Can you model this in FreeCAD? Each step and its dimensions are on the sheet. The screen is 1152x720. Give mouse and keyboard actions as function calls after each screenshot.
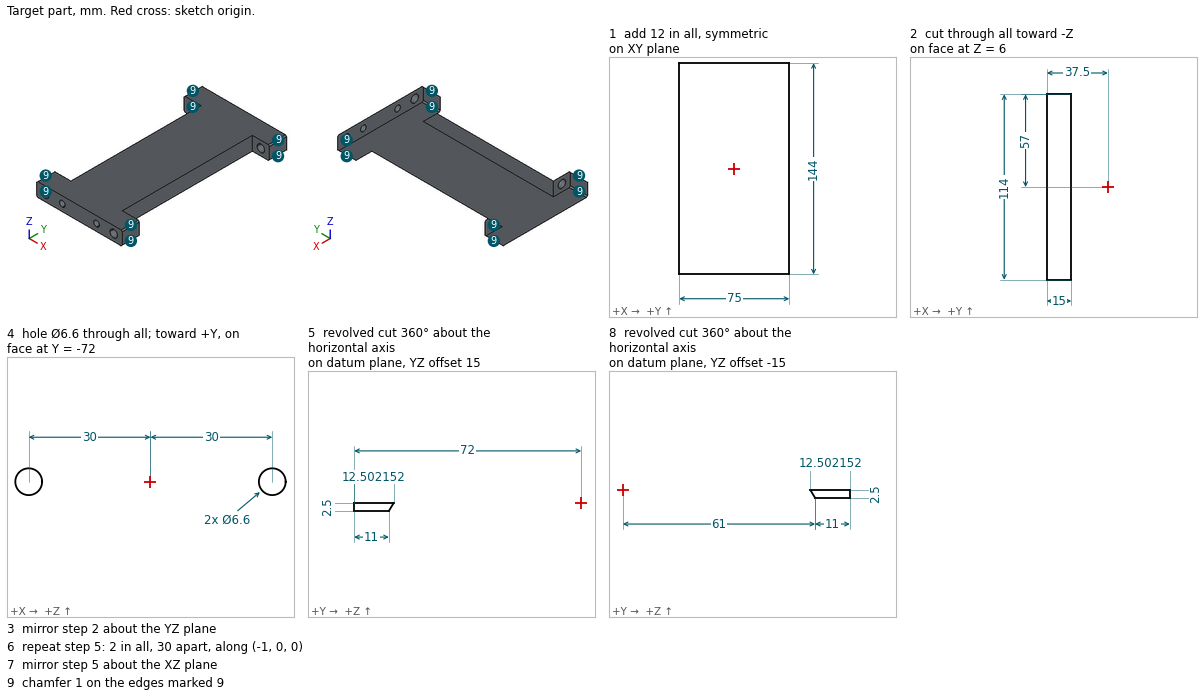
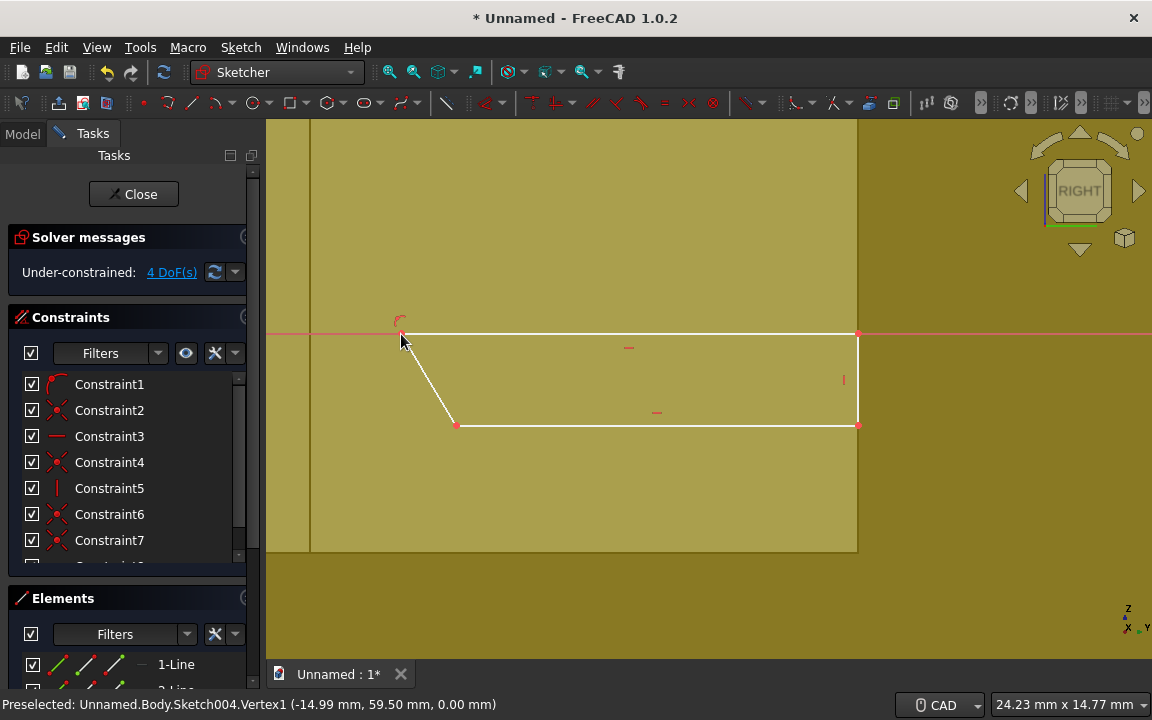
click(486, 104)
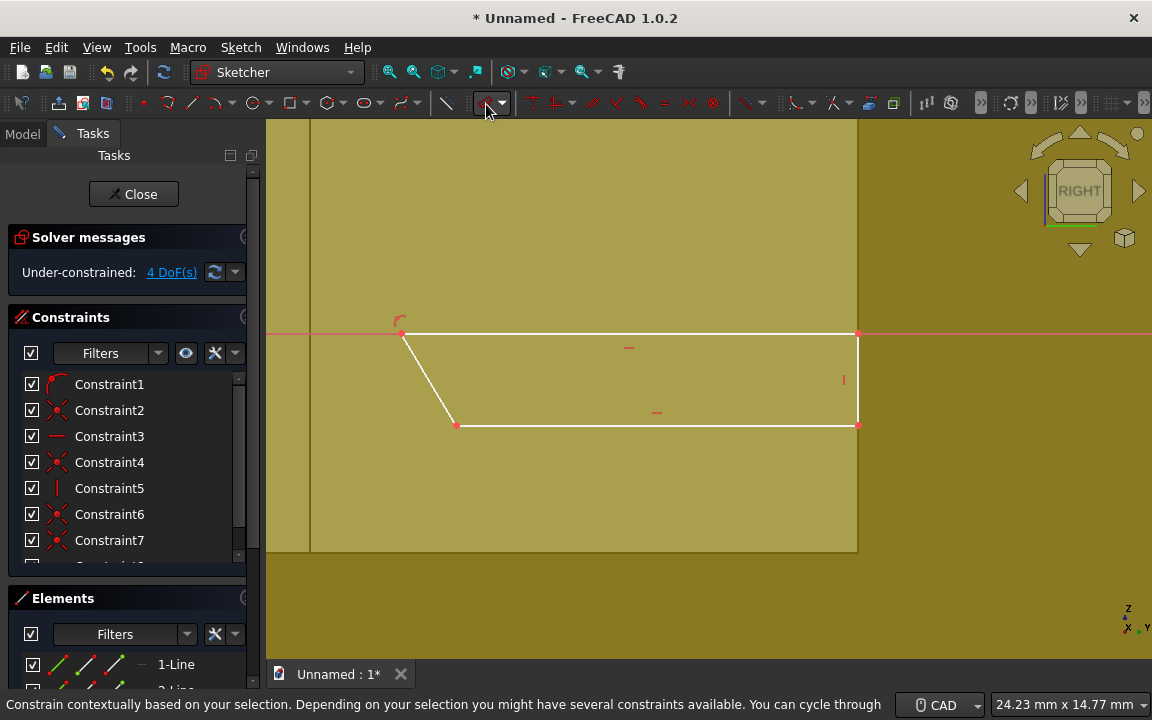
click(577, 426)
click(657, 460)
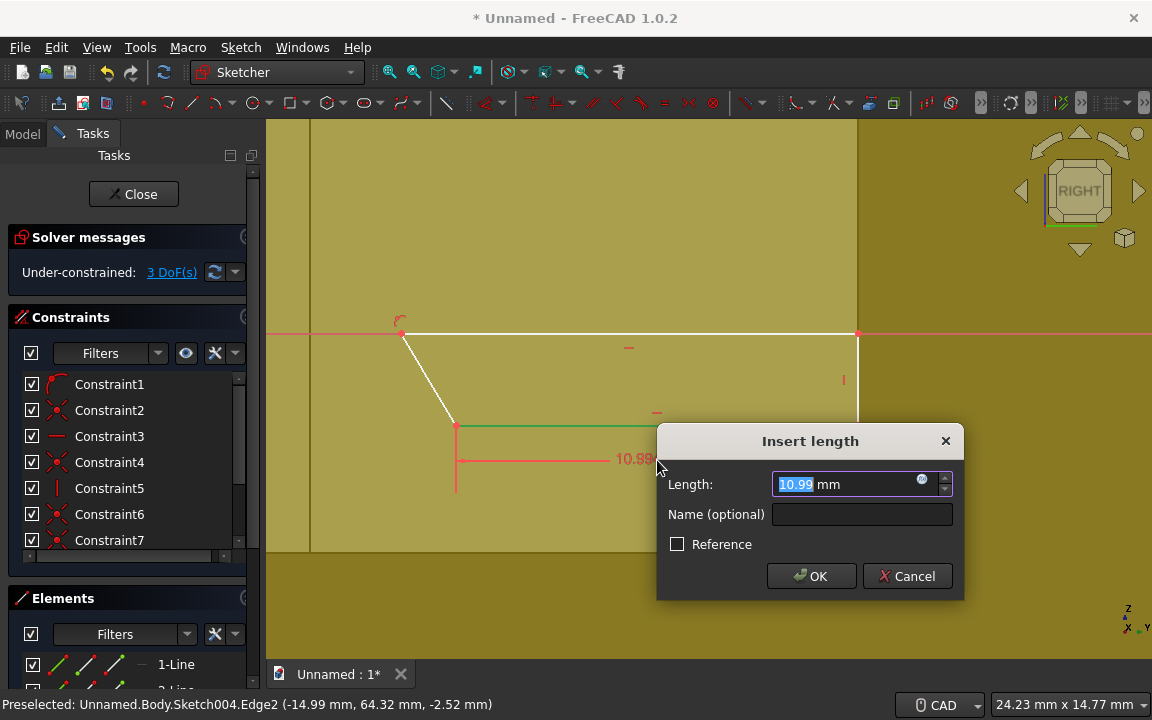
text(11)
key(Return)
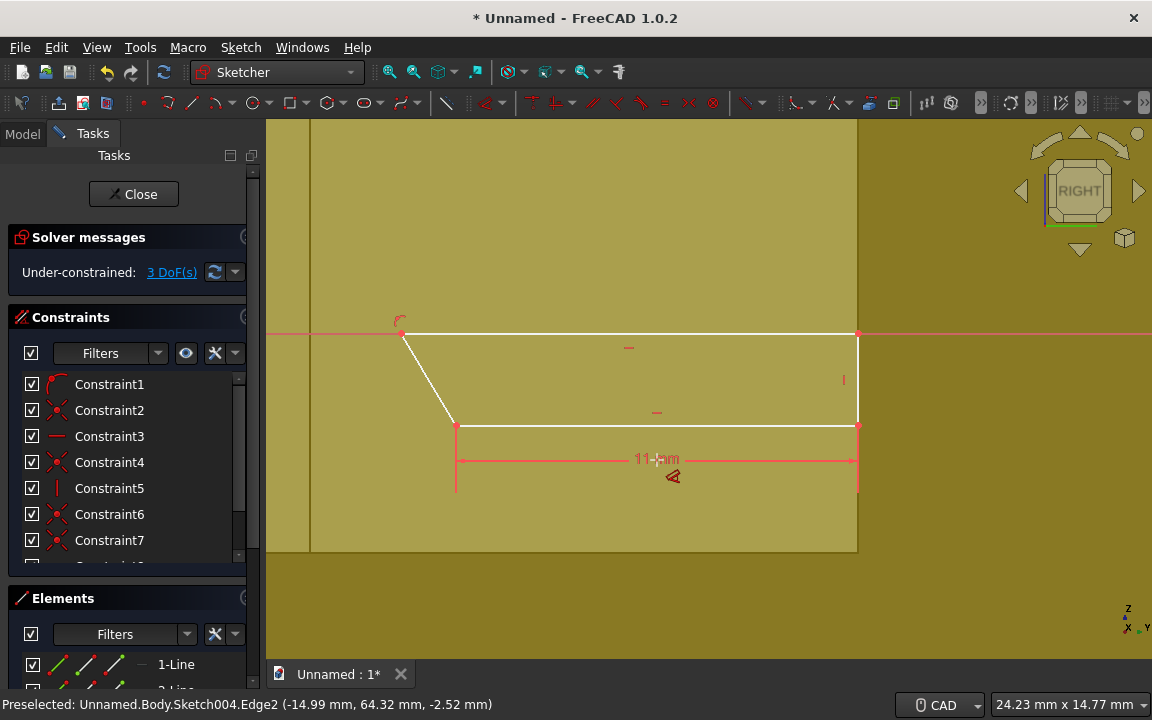
click(858, 398)
click(892, 380)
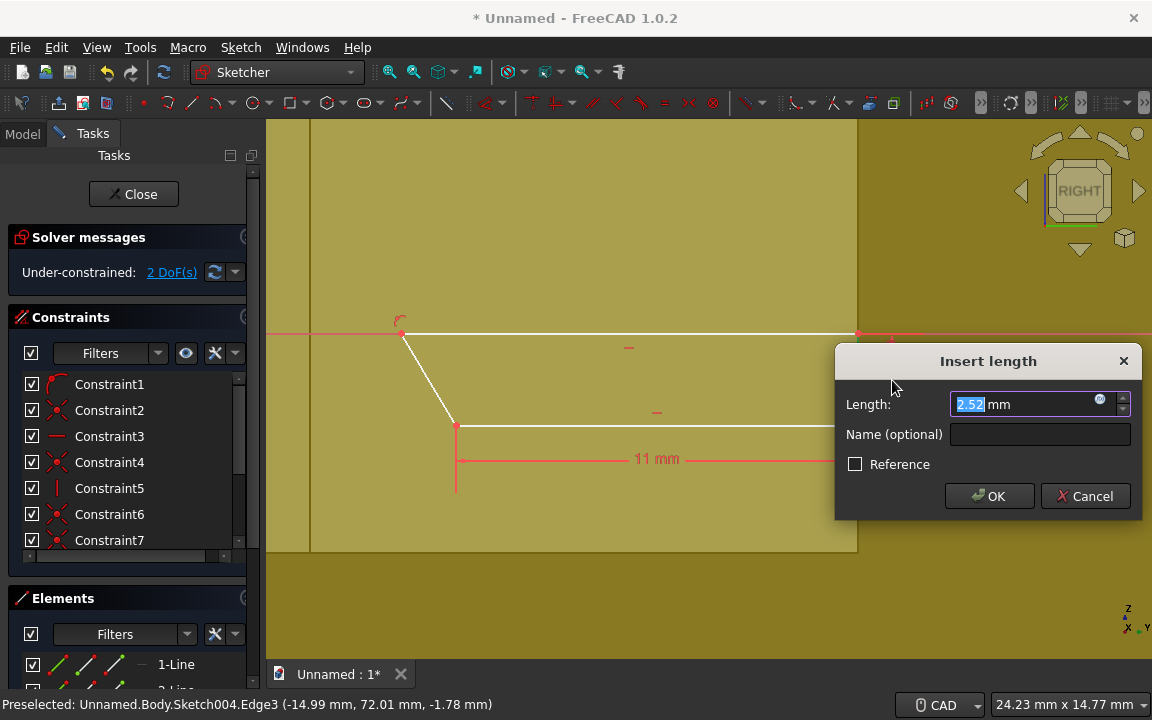
text(2.5)
key(Return)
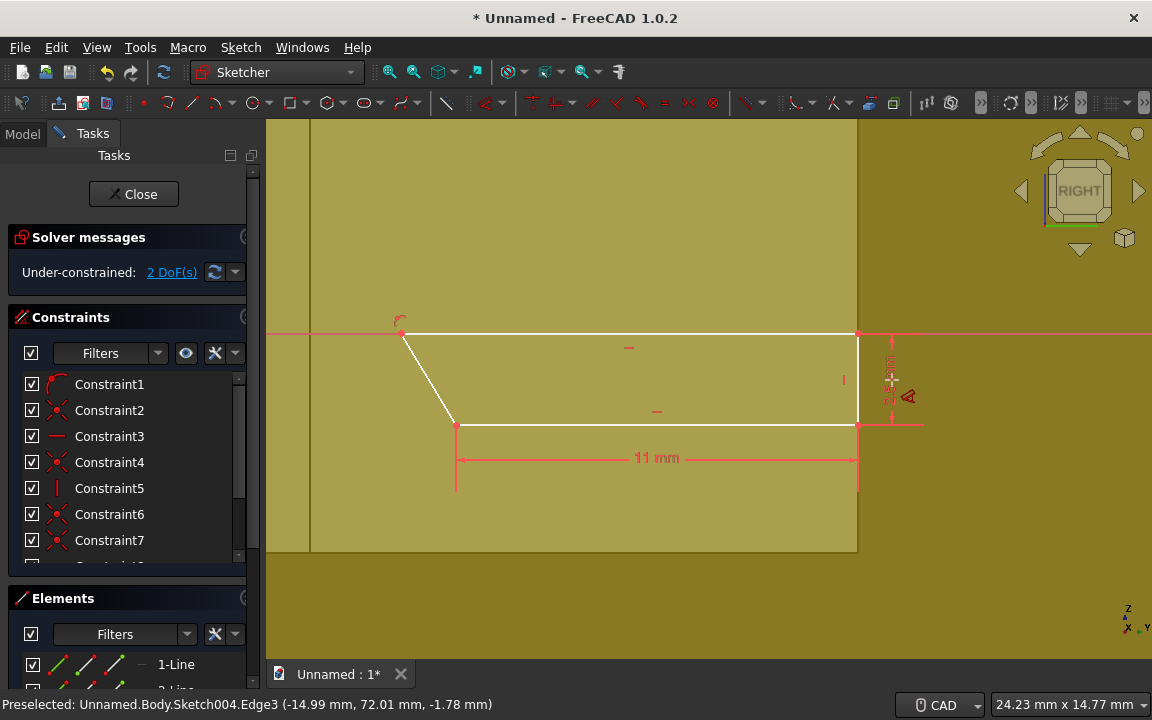
click(456, 425)
click(375, 459)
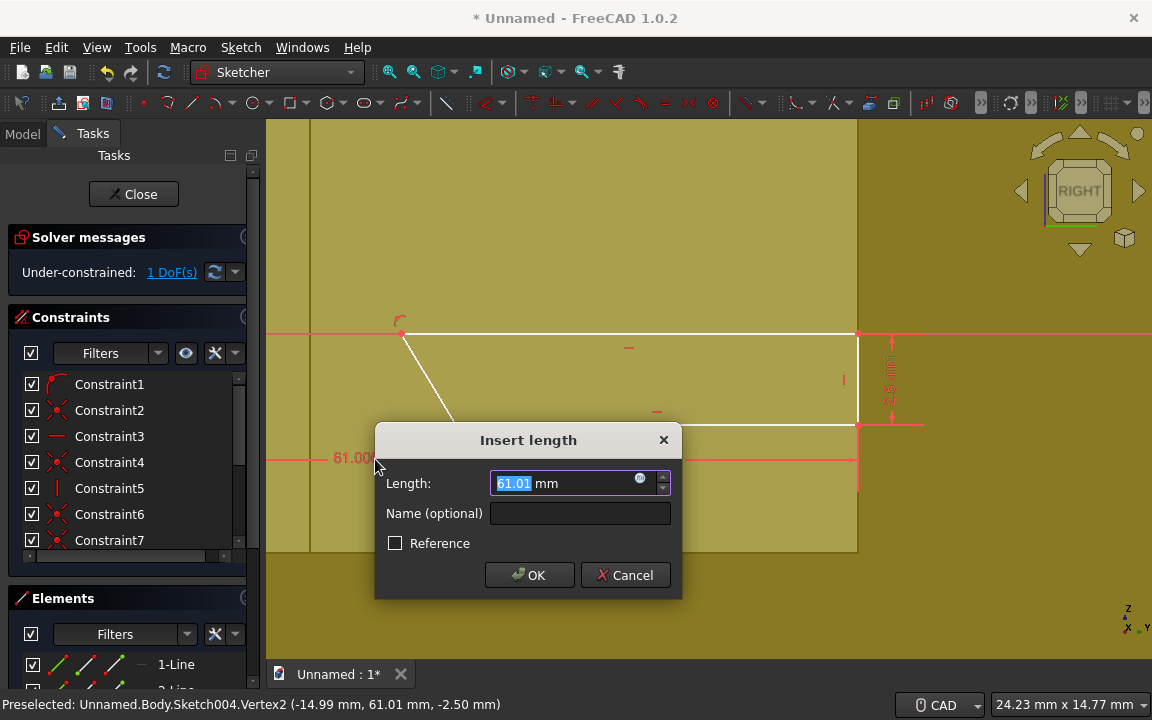
text(61)
key(Return)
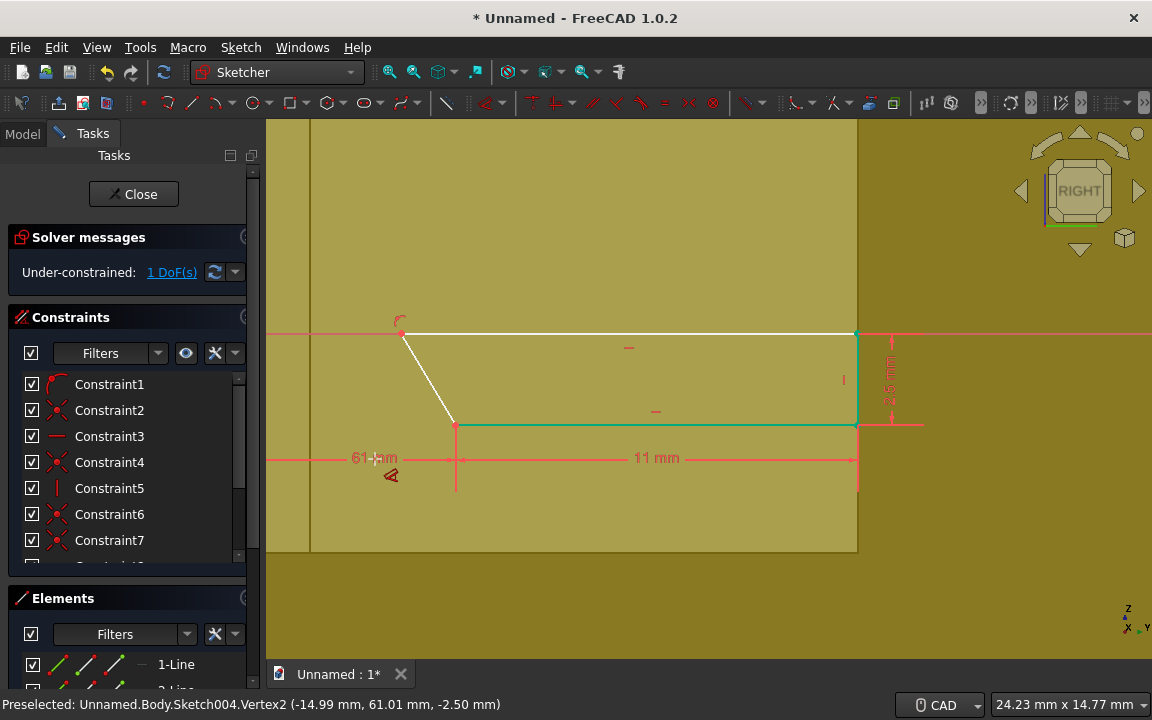
click(721, 334)
click(629, 300)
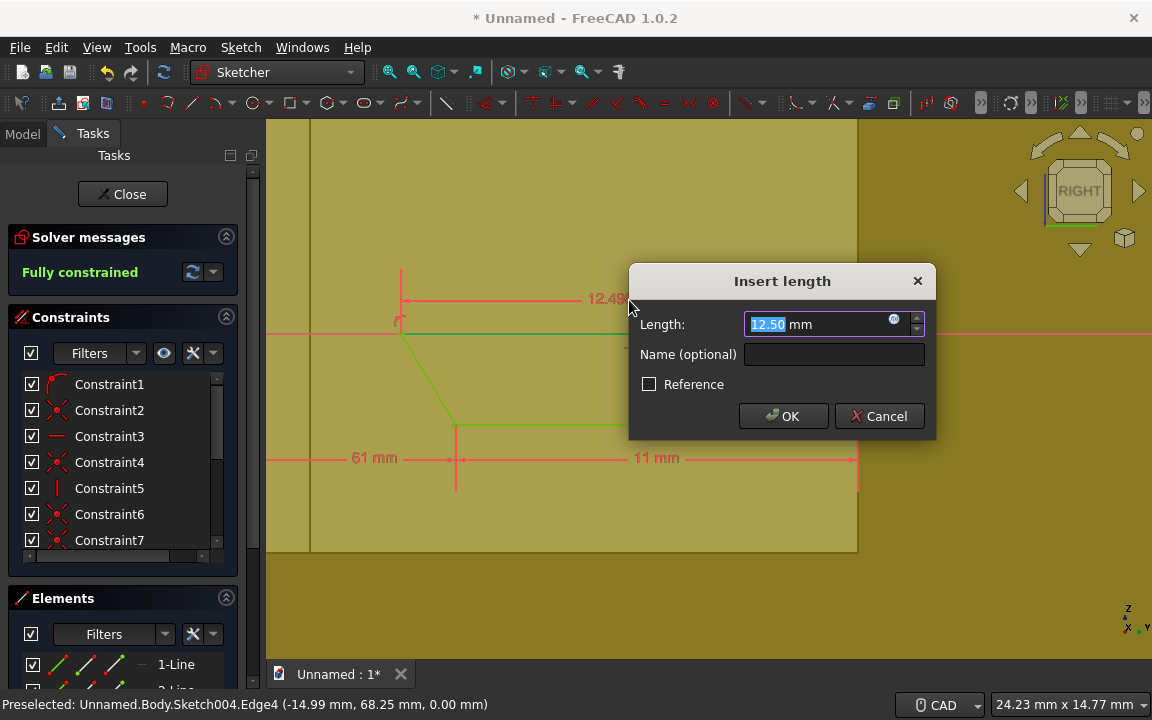
text(12.502152)
key(Return)
key(Escape)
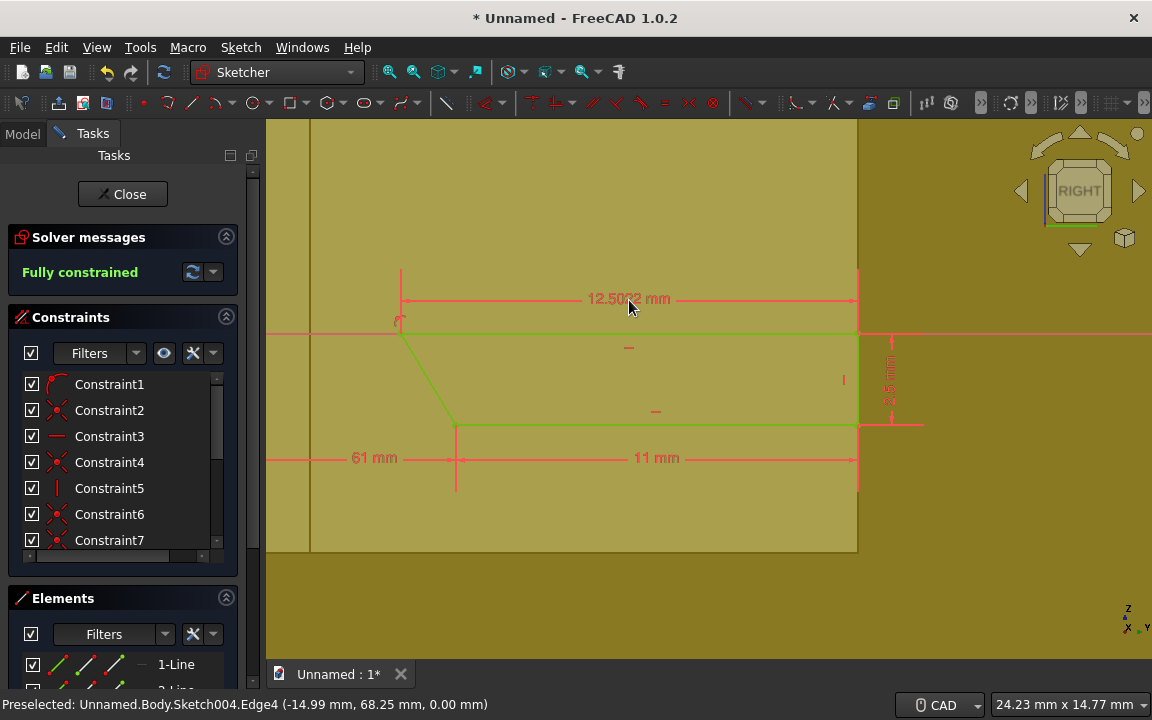
click(123, 194)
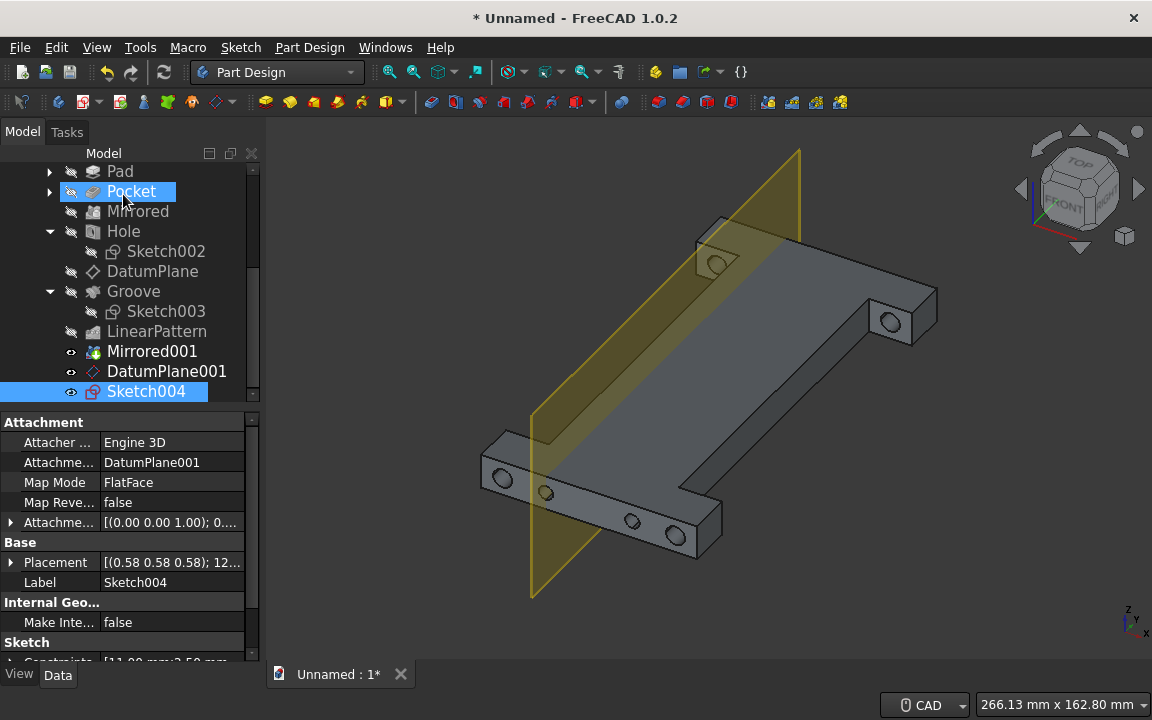
click(480, 102)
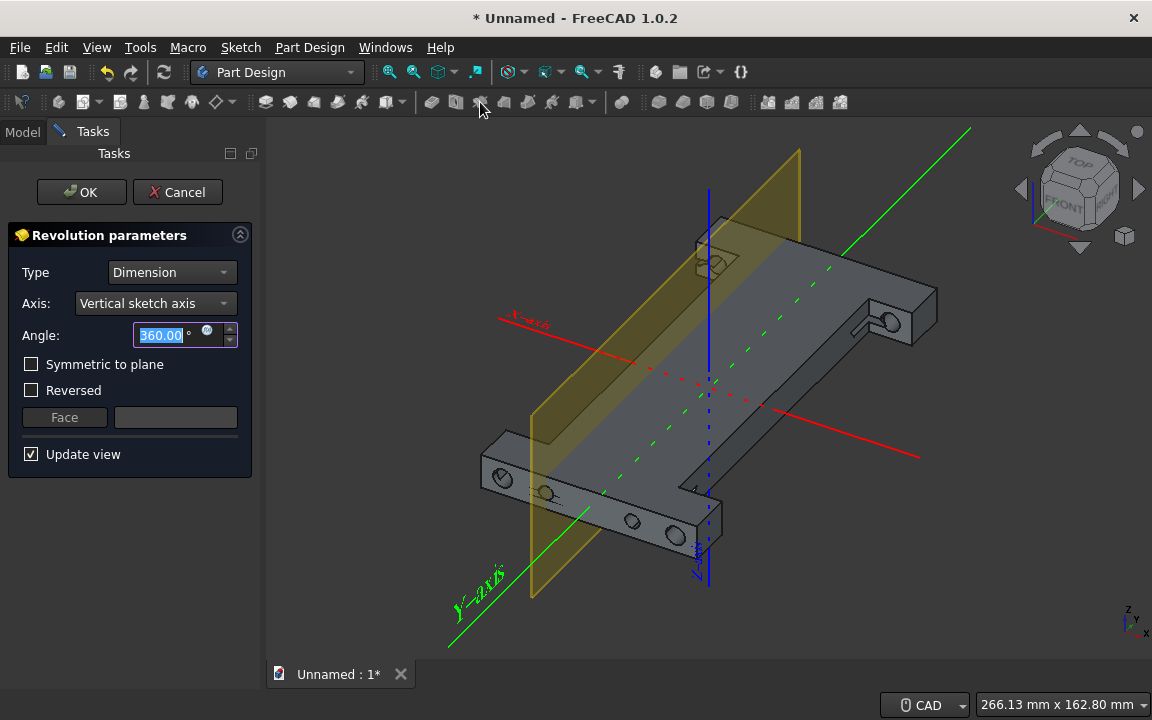
click(156, 304)